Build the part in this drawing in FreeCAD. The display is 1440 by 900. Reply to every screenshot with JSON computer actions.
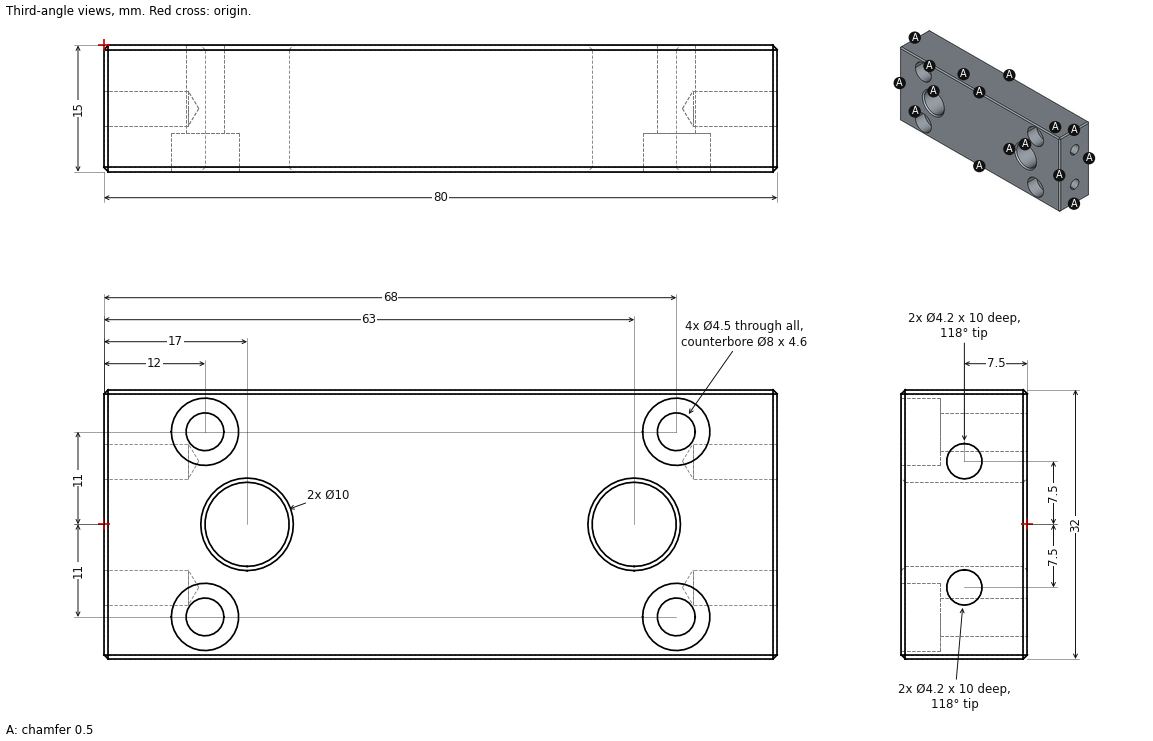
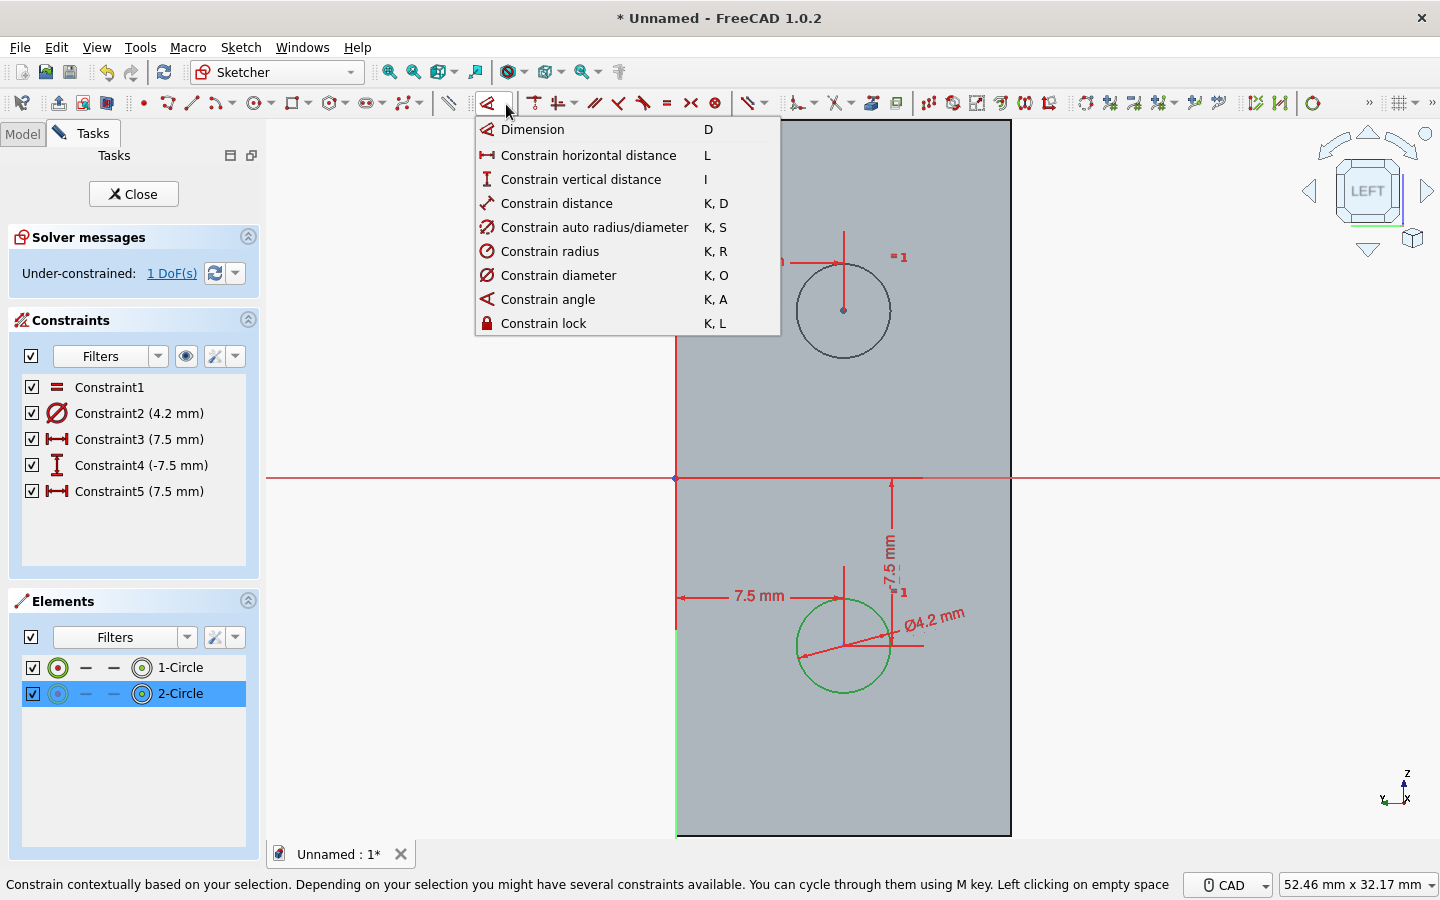
{"action": "left_click", "coordinate": [628, 179]}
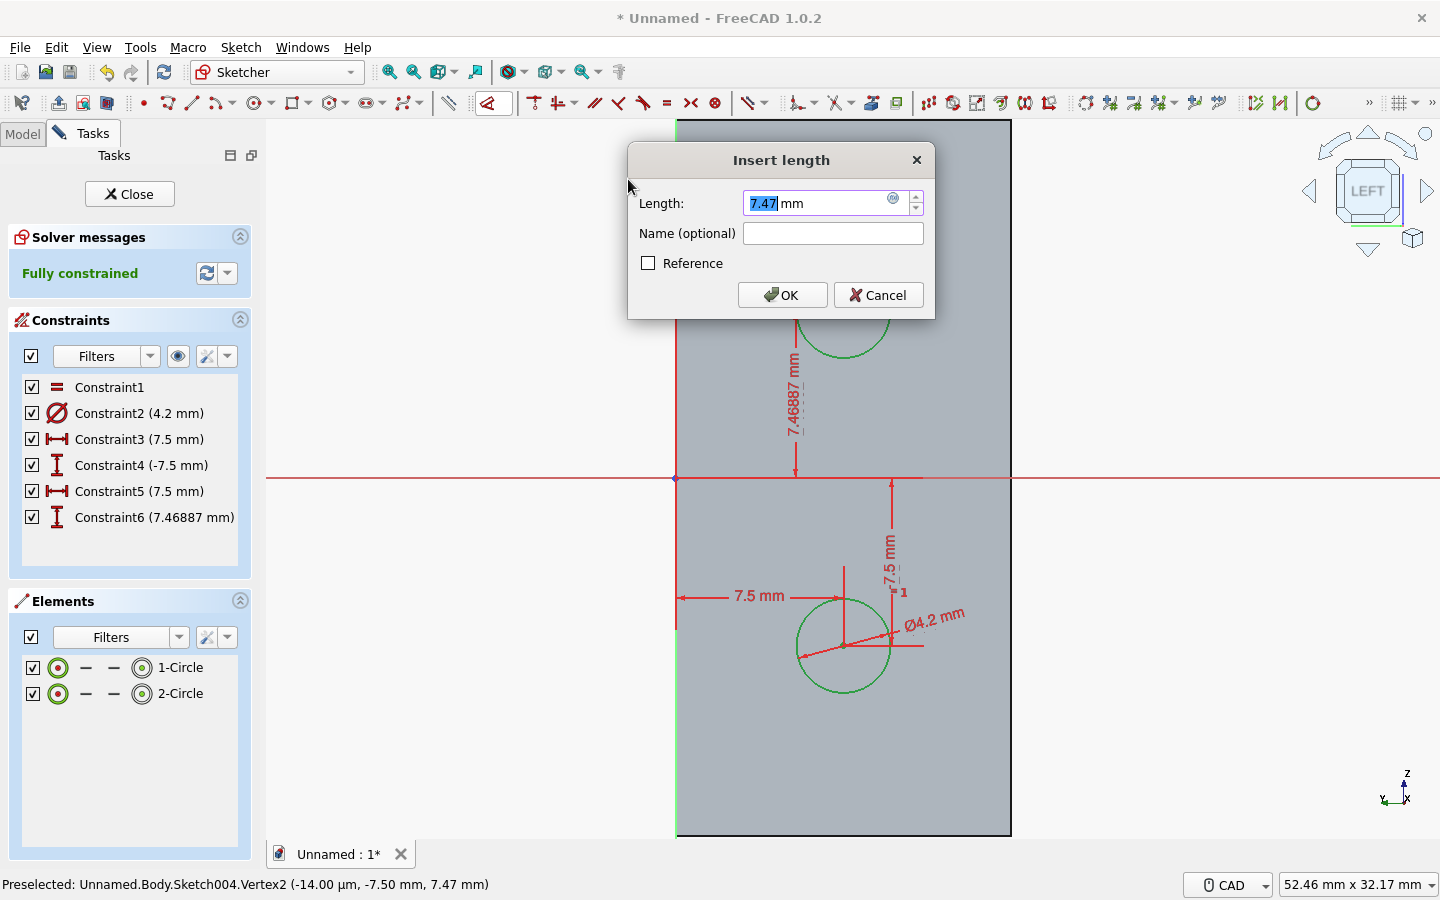
{"action": "type", "text": "7.5"}
{"action": "key", "text": "Return"}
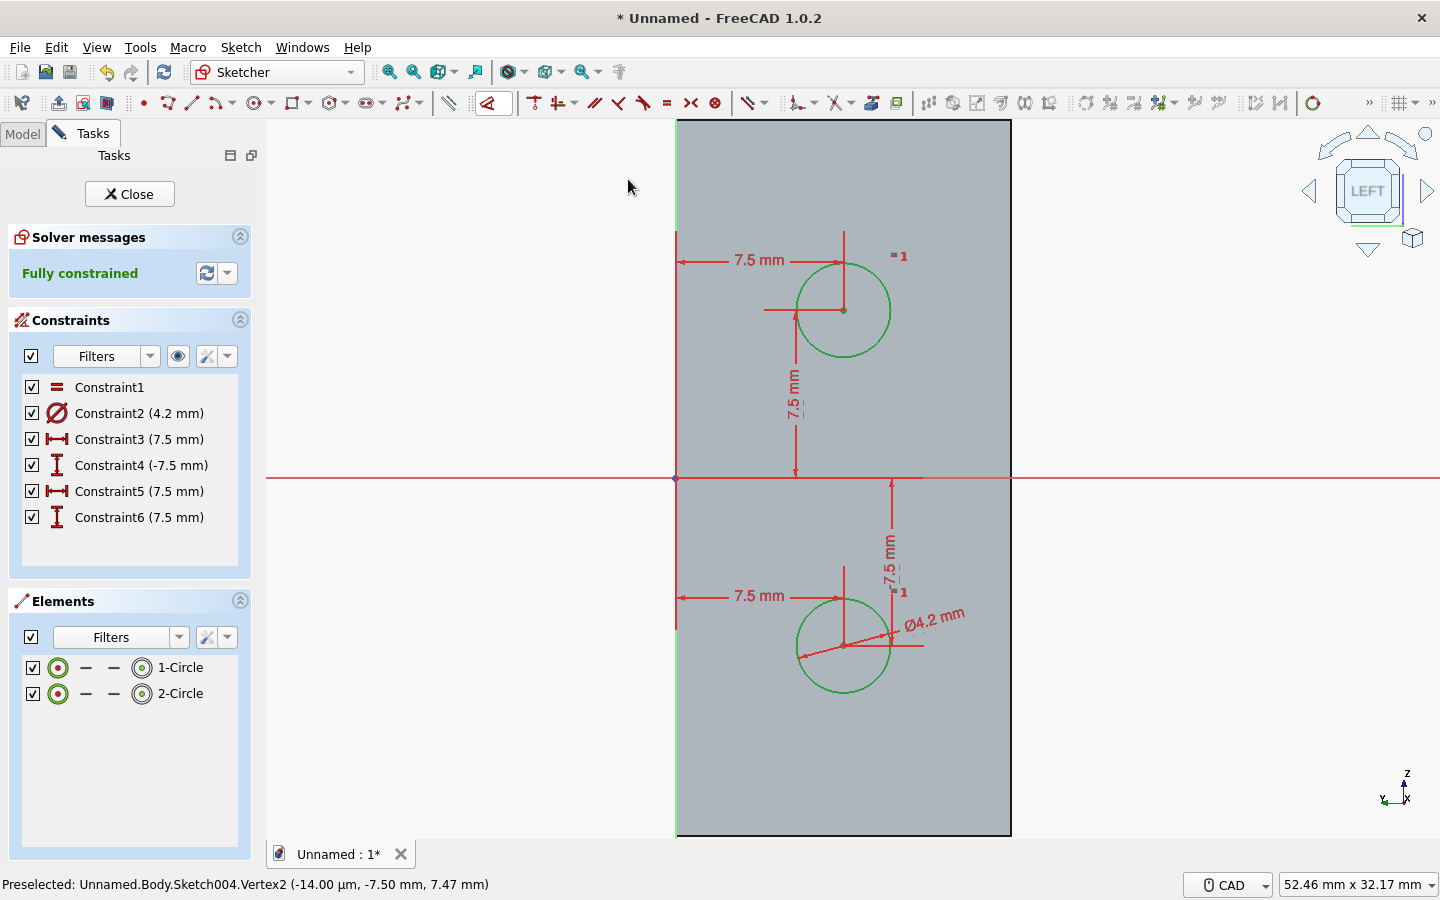
{"action": "left_click", "coordinate": [130, 194]}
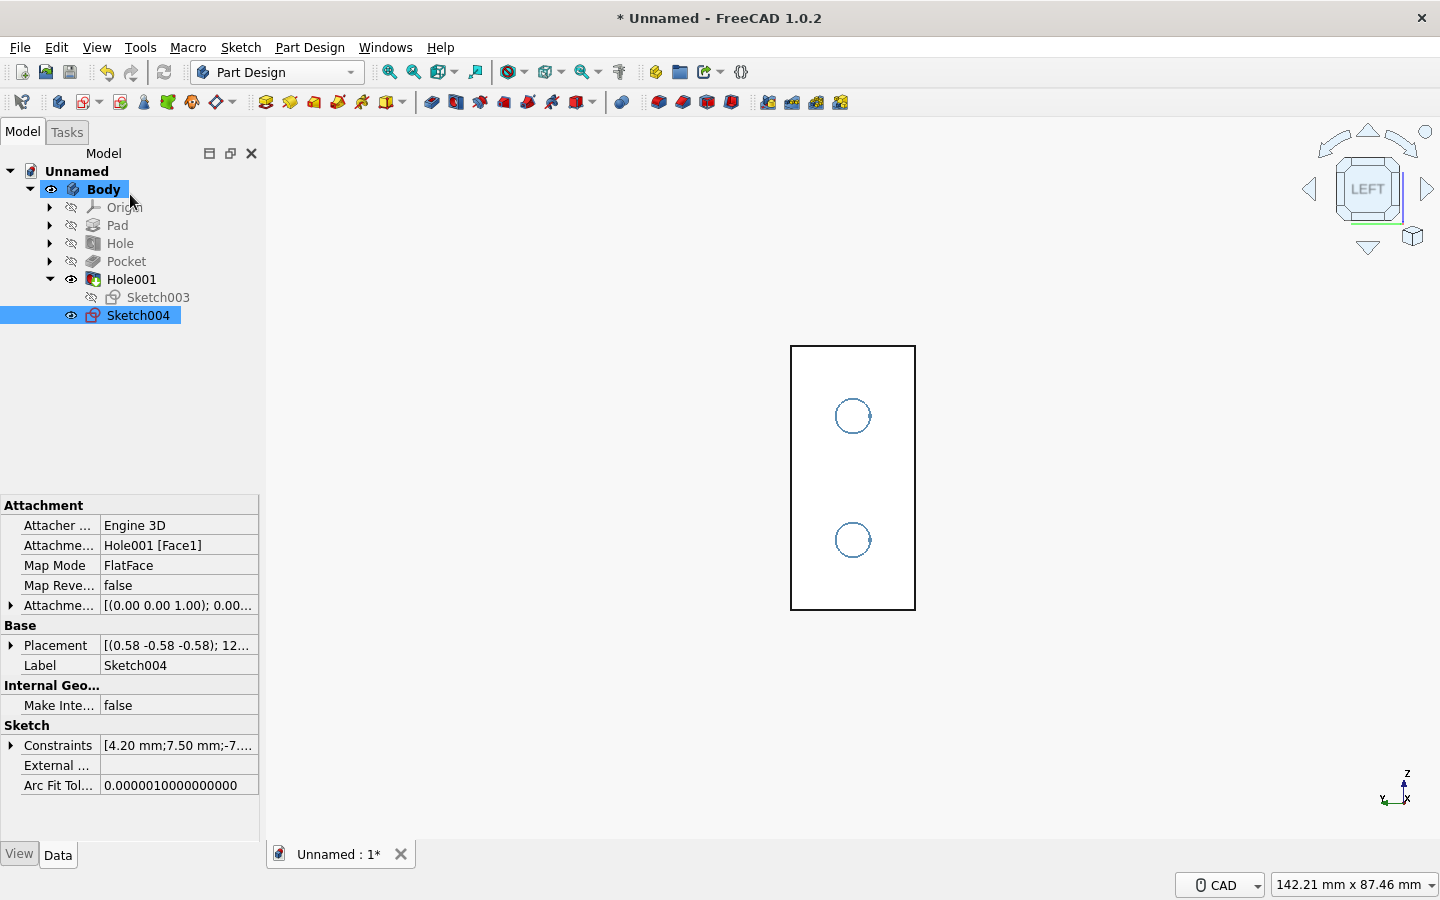
{"action": "left_click", "coordinate": [456, 102]}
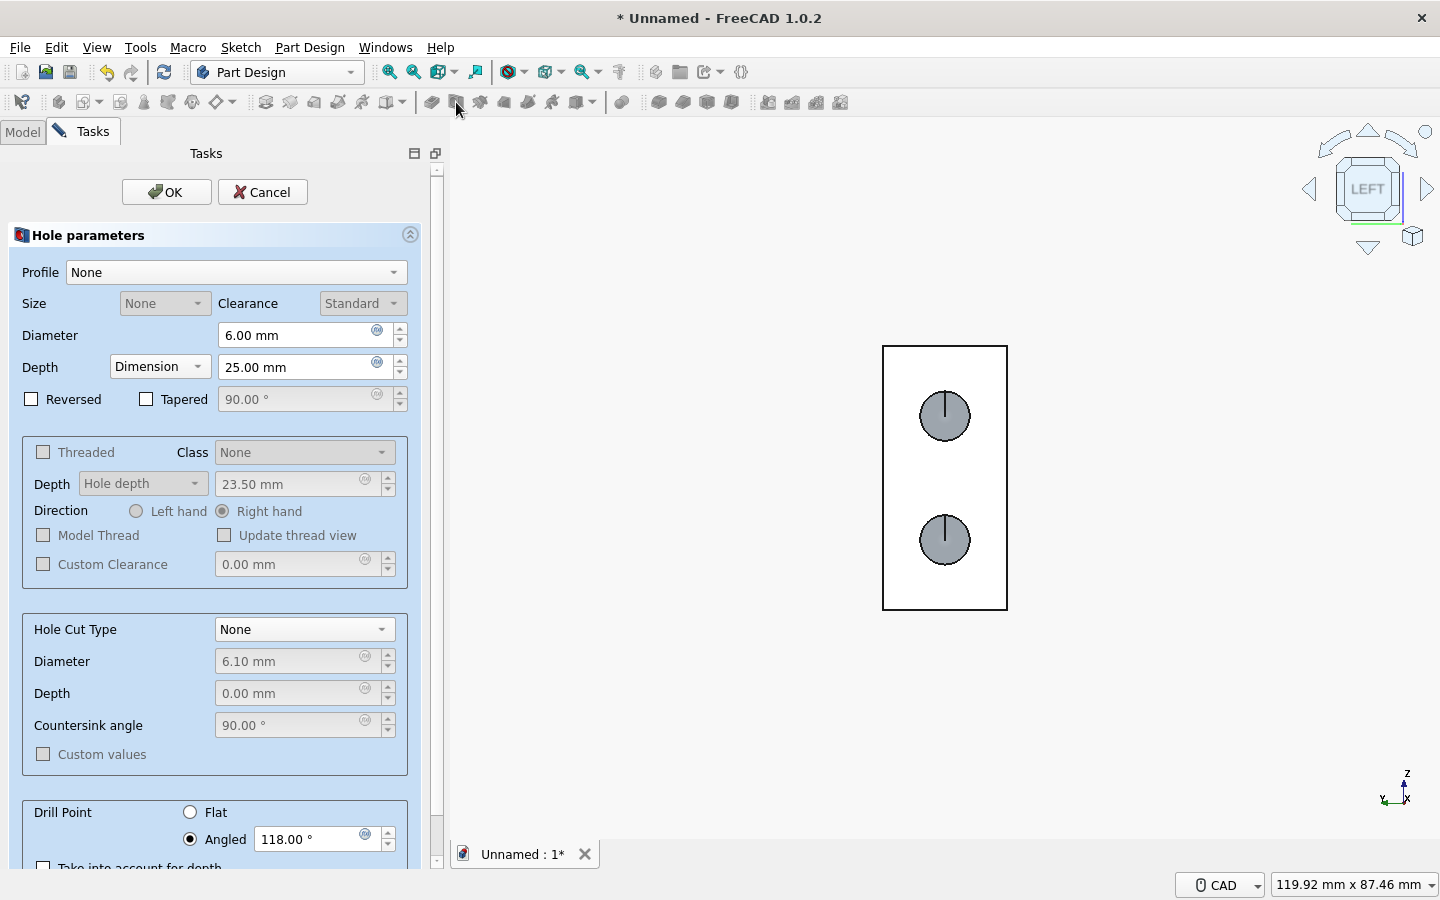
{"action": "triple_click", "coordinate": [305, 335]}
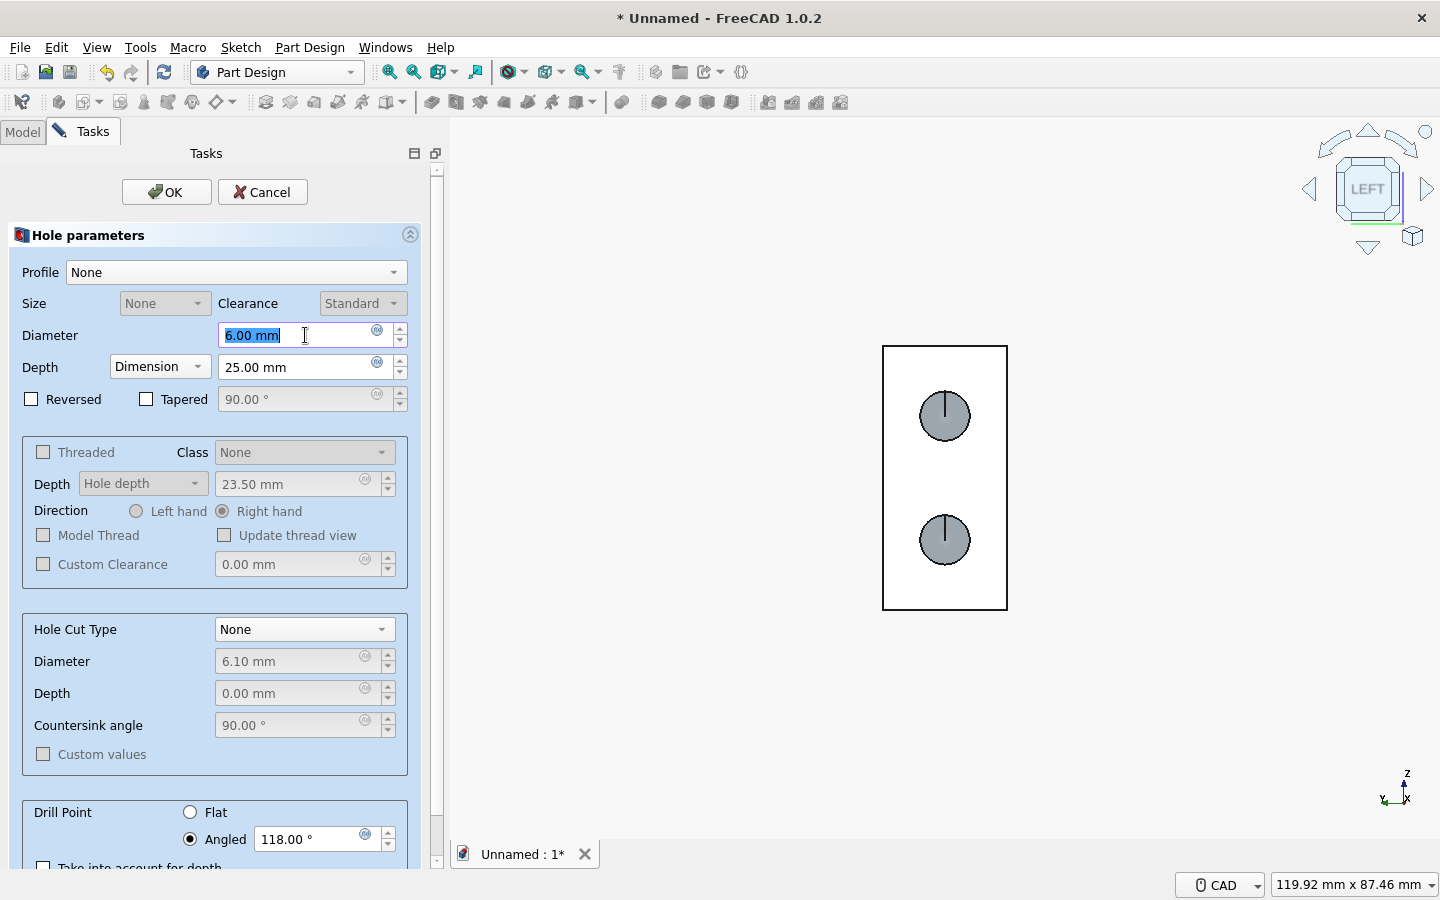
{"action": "type", "text": "4.2"}
{"action": "key", "text": "Tab"}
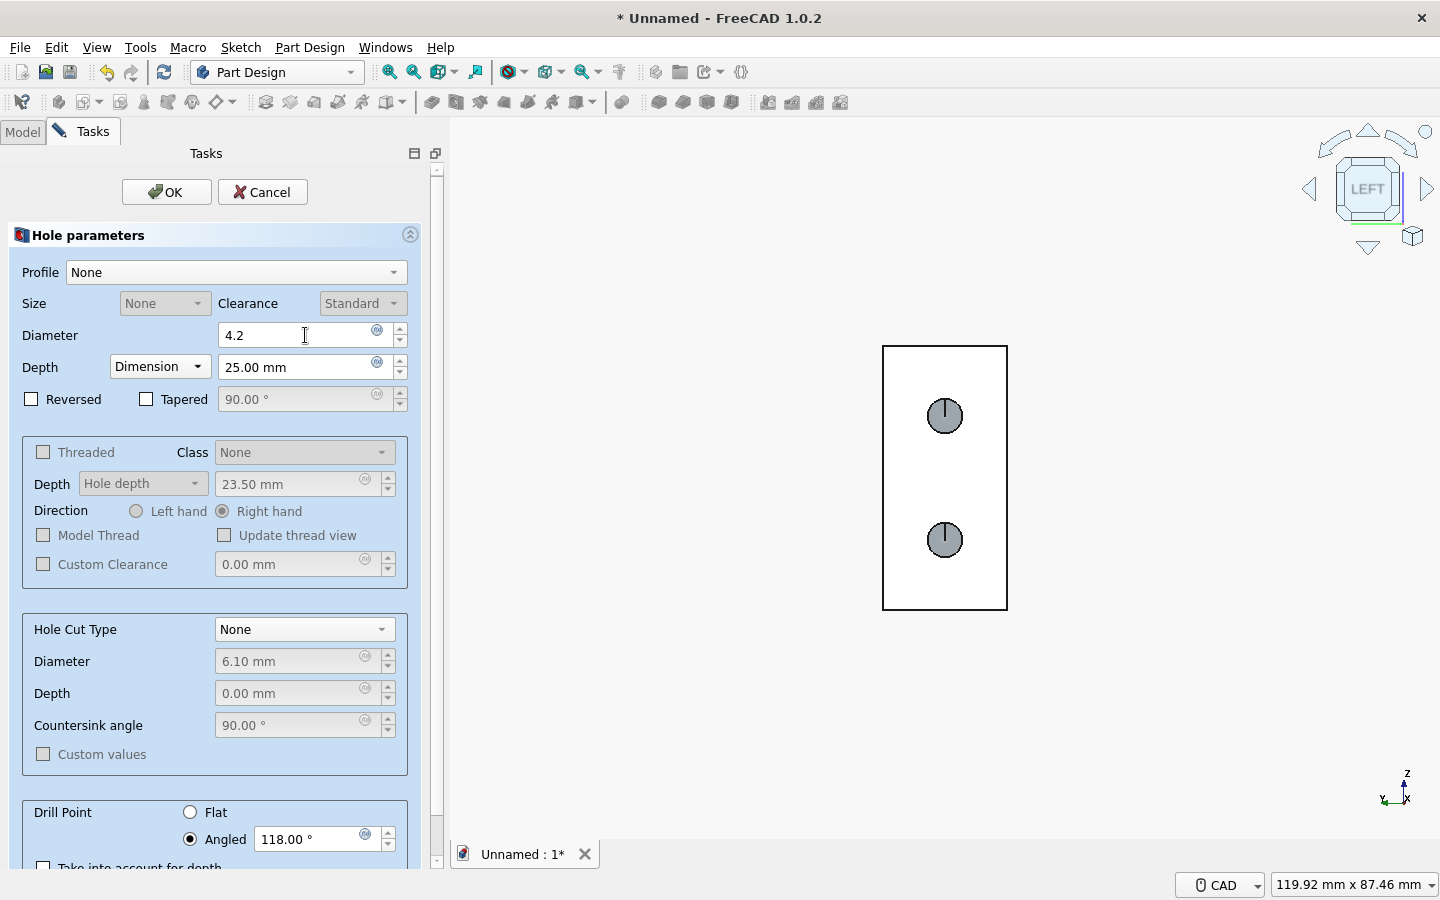
{"action": "triple_click", "coordinate": [305, 367]}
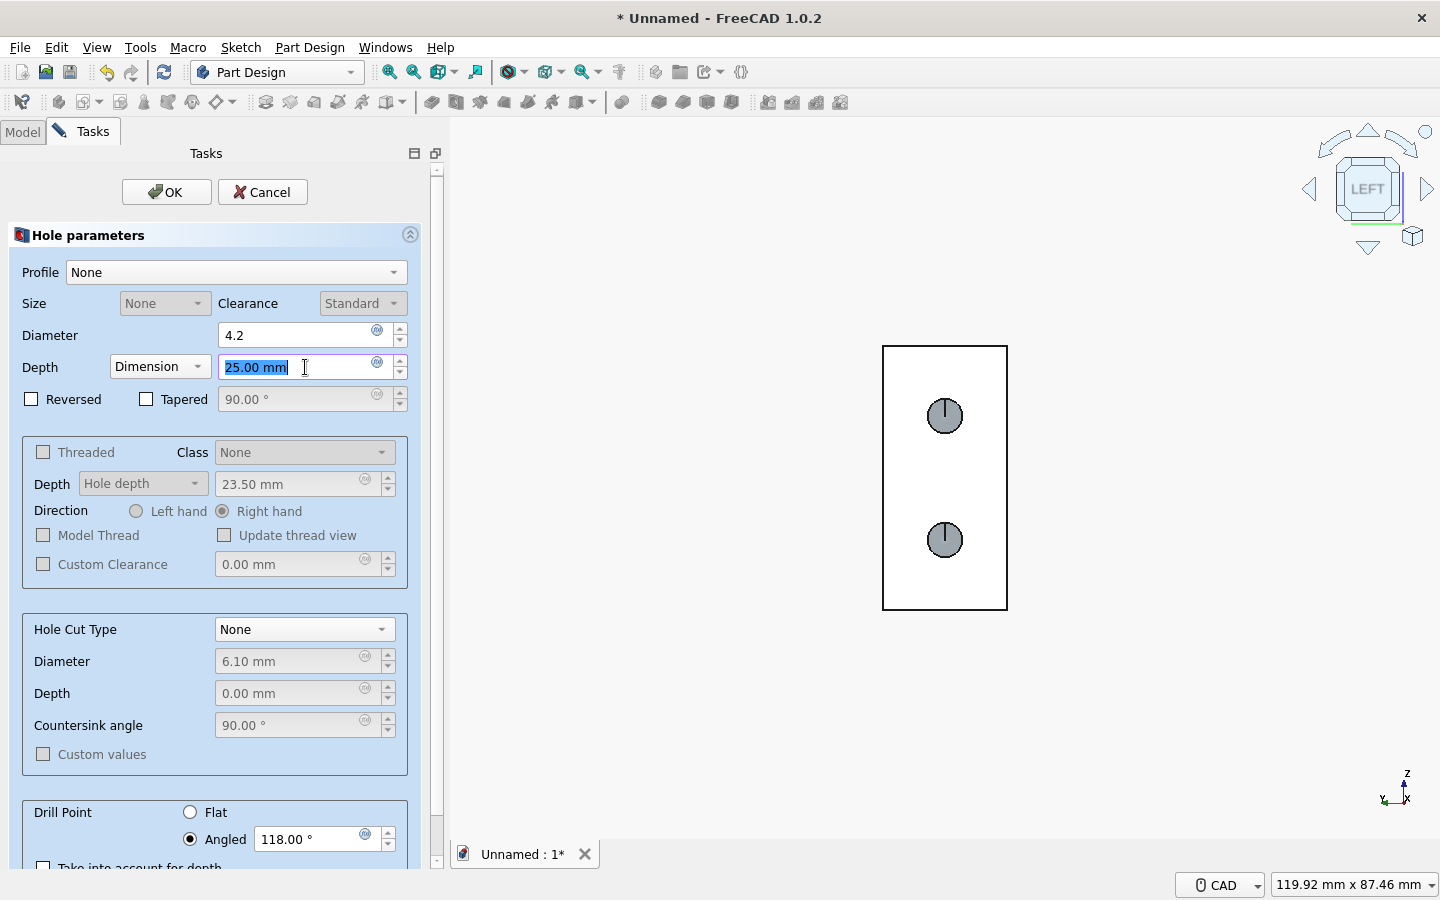
{"action": "type", "text": "10"}
{"action": "key", "text": "Tab"}